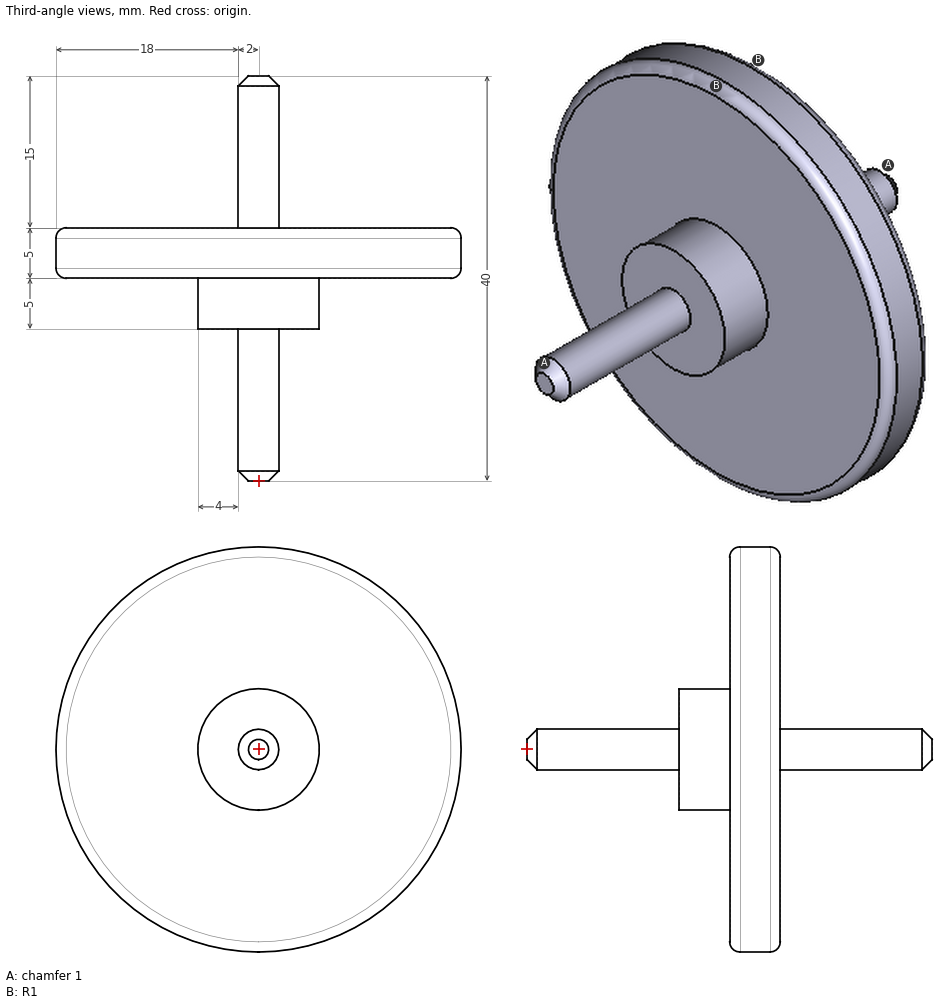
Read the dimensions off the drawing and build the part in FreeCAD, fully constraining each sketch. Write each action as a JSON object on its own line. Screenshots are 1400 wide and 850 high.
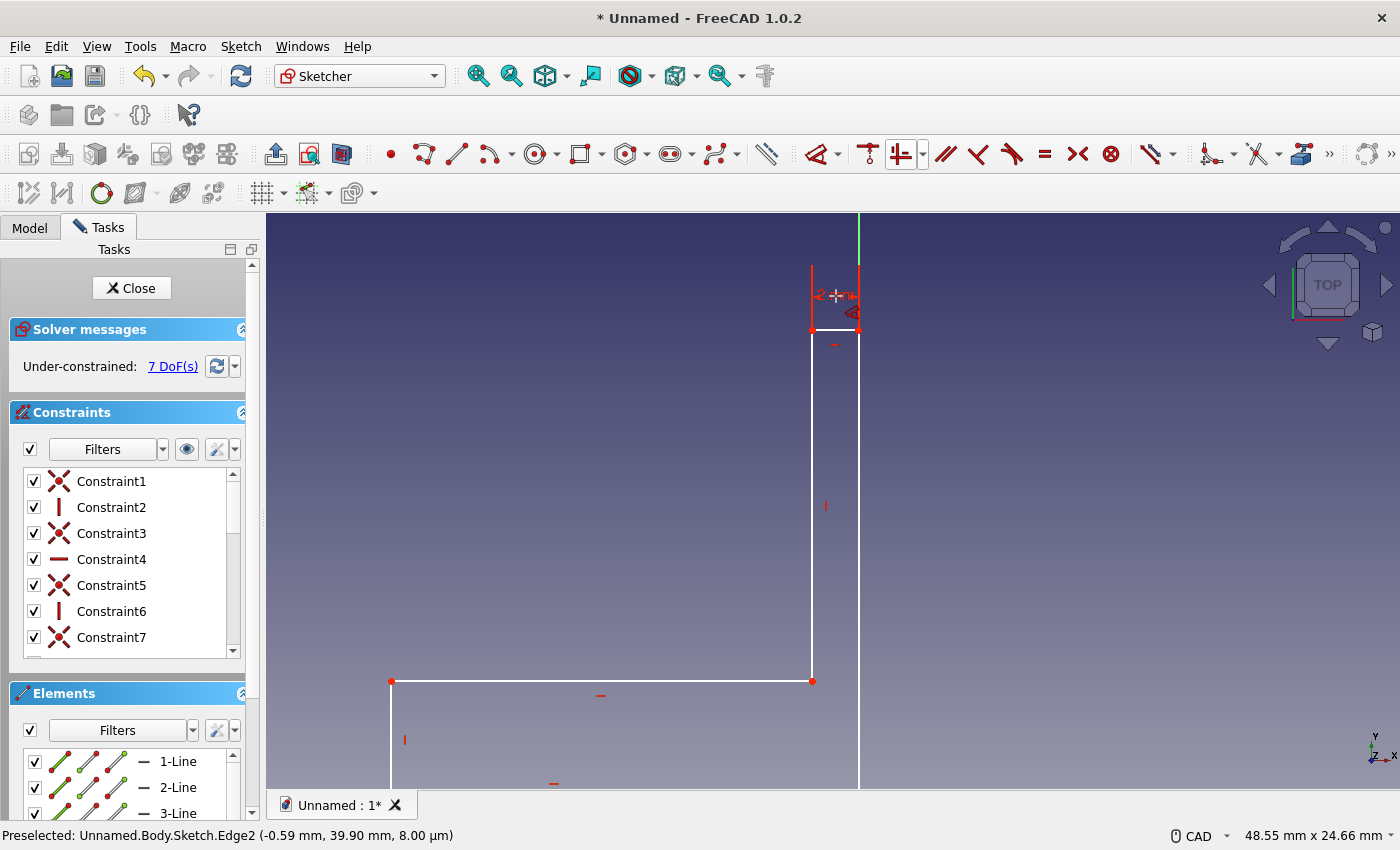
{"action": "left_click", "coordinate": [391, 716]}
{"action": "left_click", "coordinate": [357, 721]}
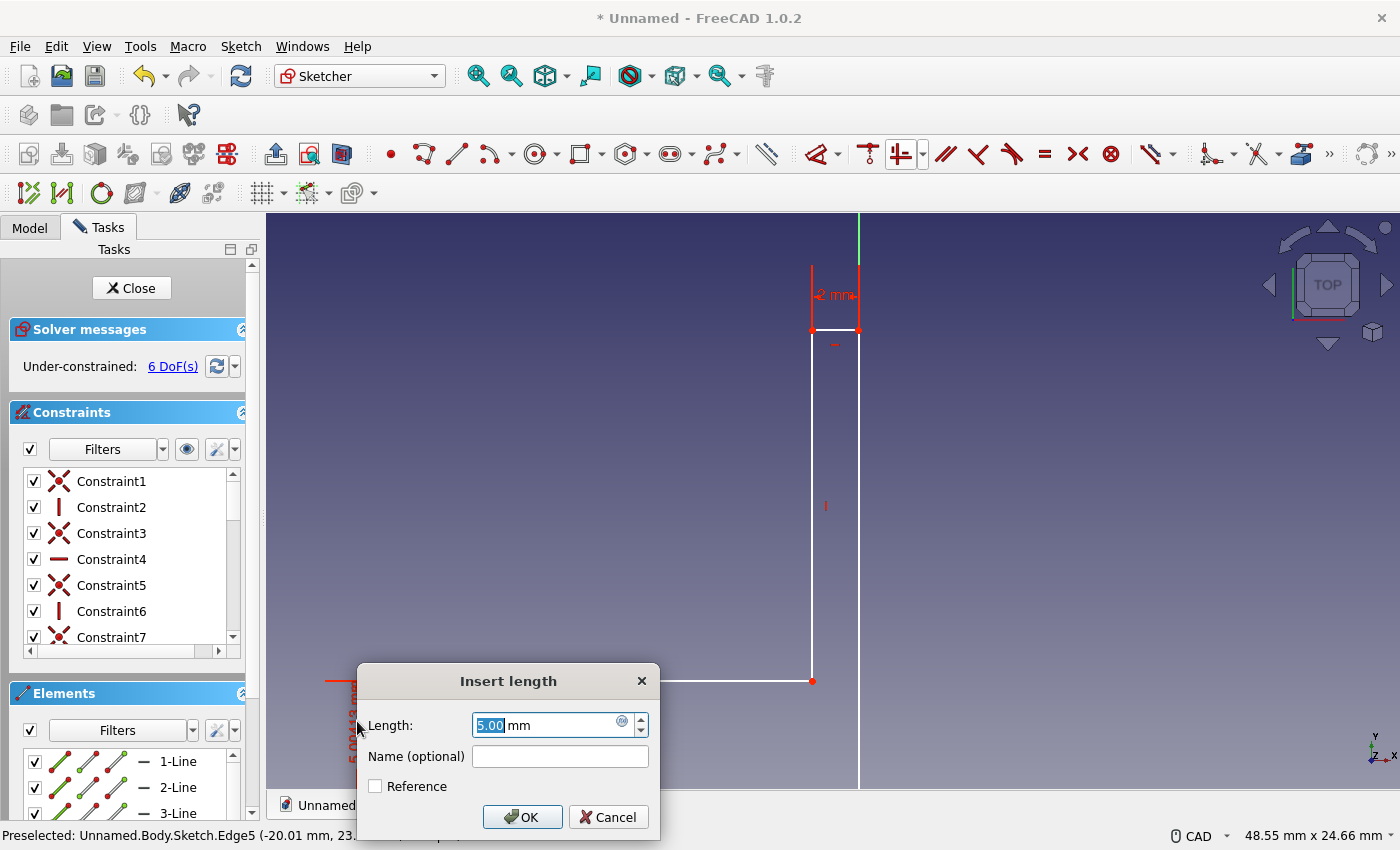
{"action": "type", "text": "5"}
{"action": "key", "text": "Return"}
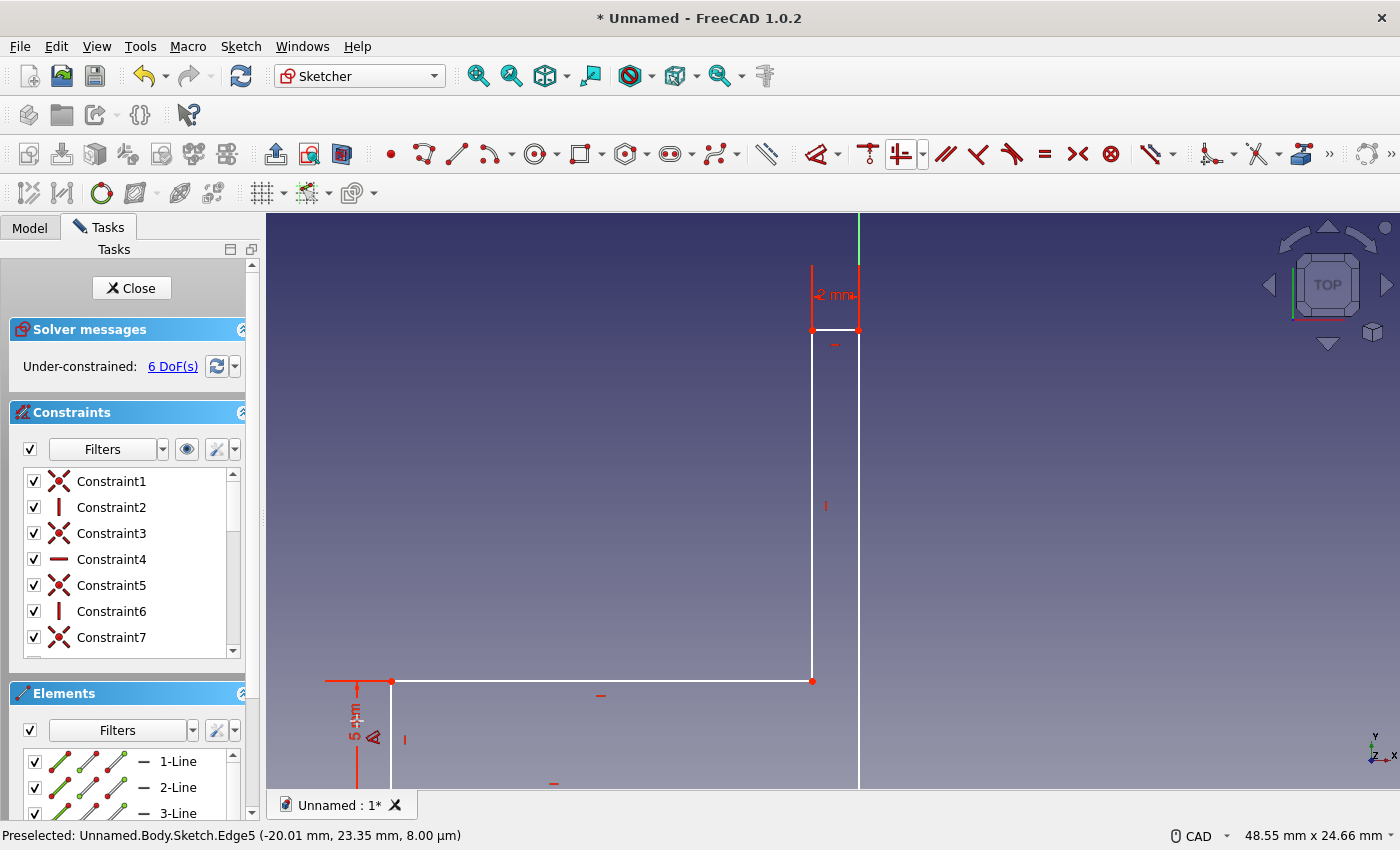
{"action": "scroll", "coordinate": [846, 330], "scroll_direction": "down", "scroll_amount": 5}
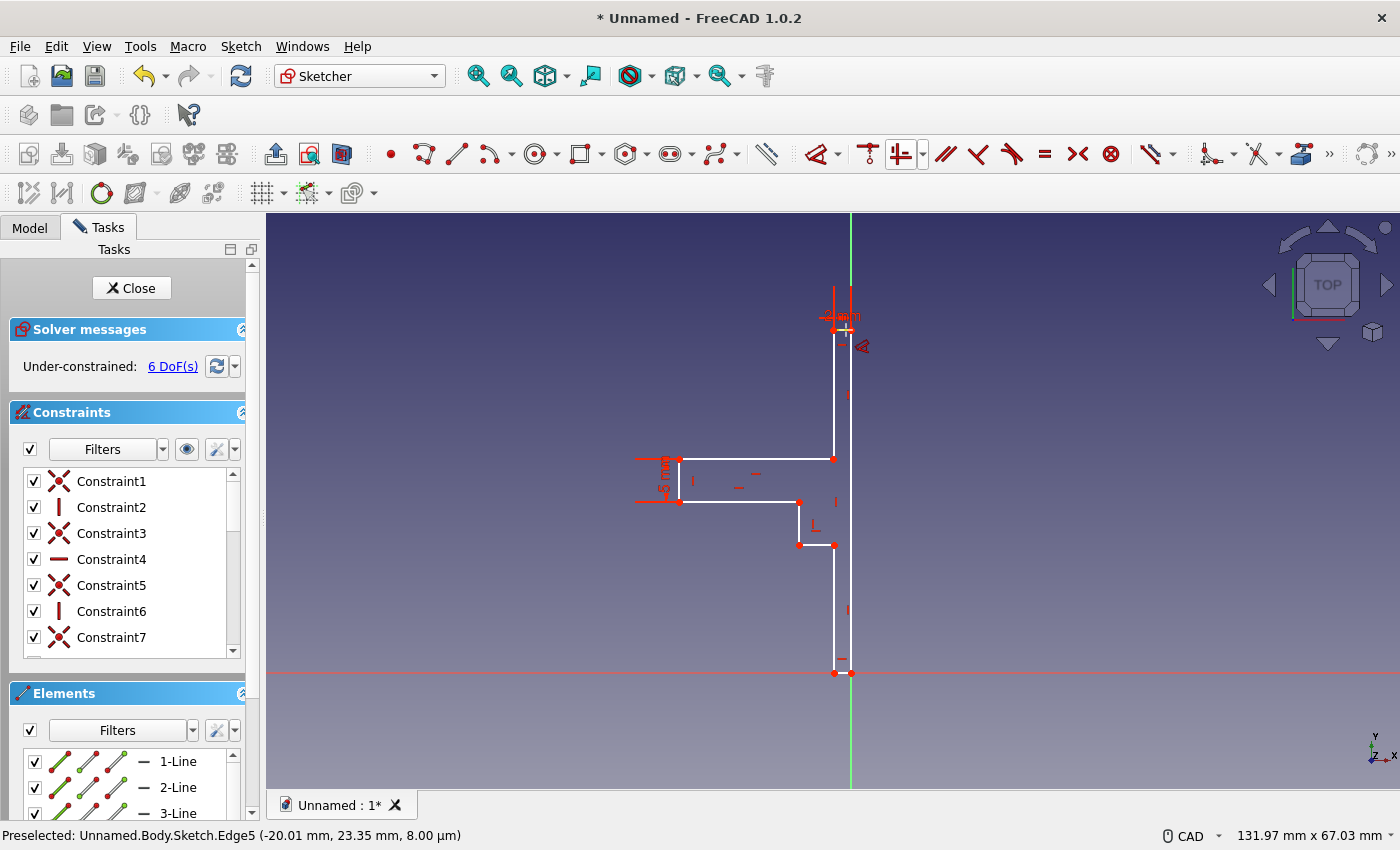
{"action": "left_click", "coordinate": [799, 515]}
{"action": "left_click", "coordinate": [833, 524]}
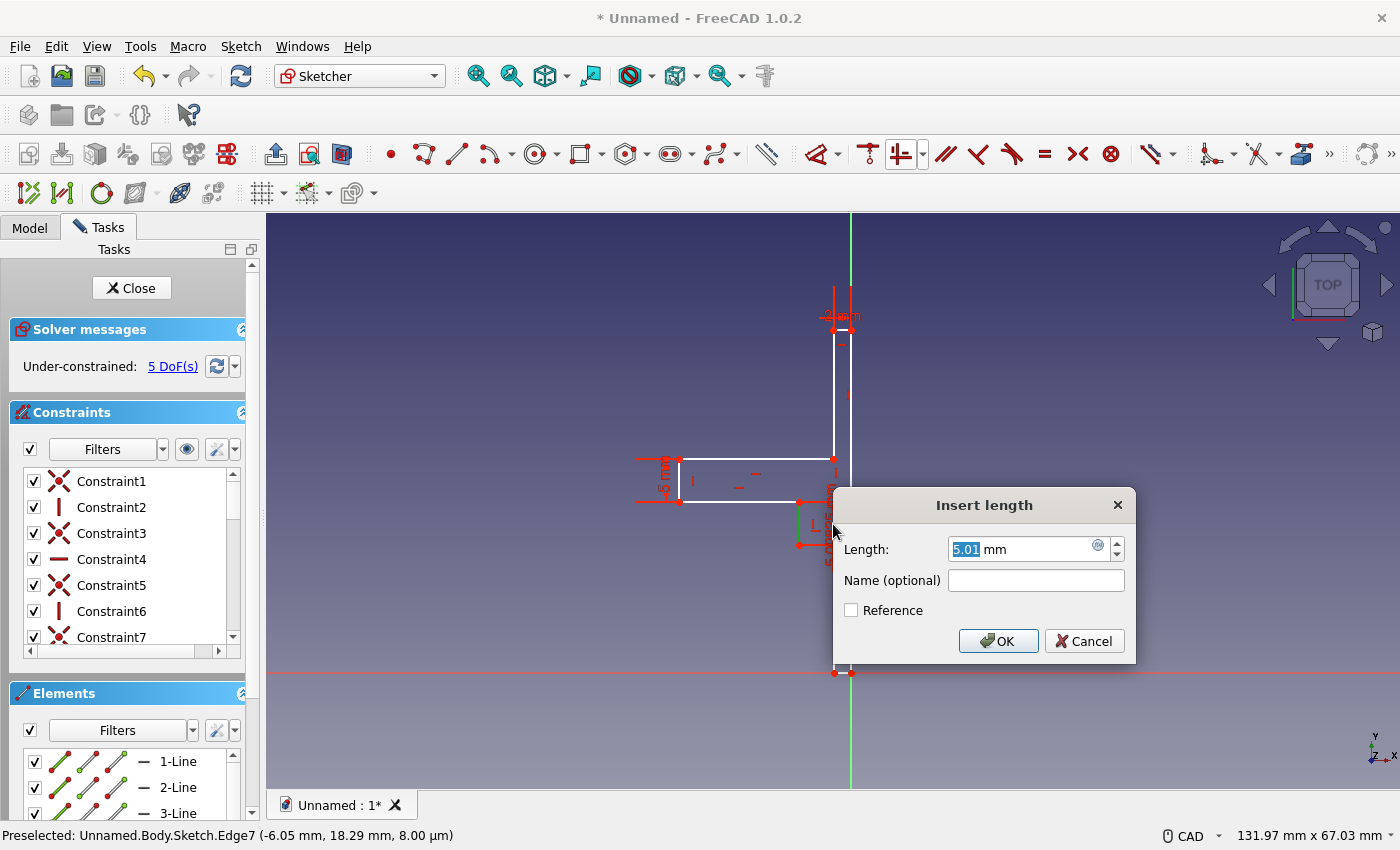
{"action": "type", "text": "5"}
{"action": "key", "text": "Return"}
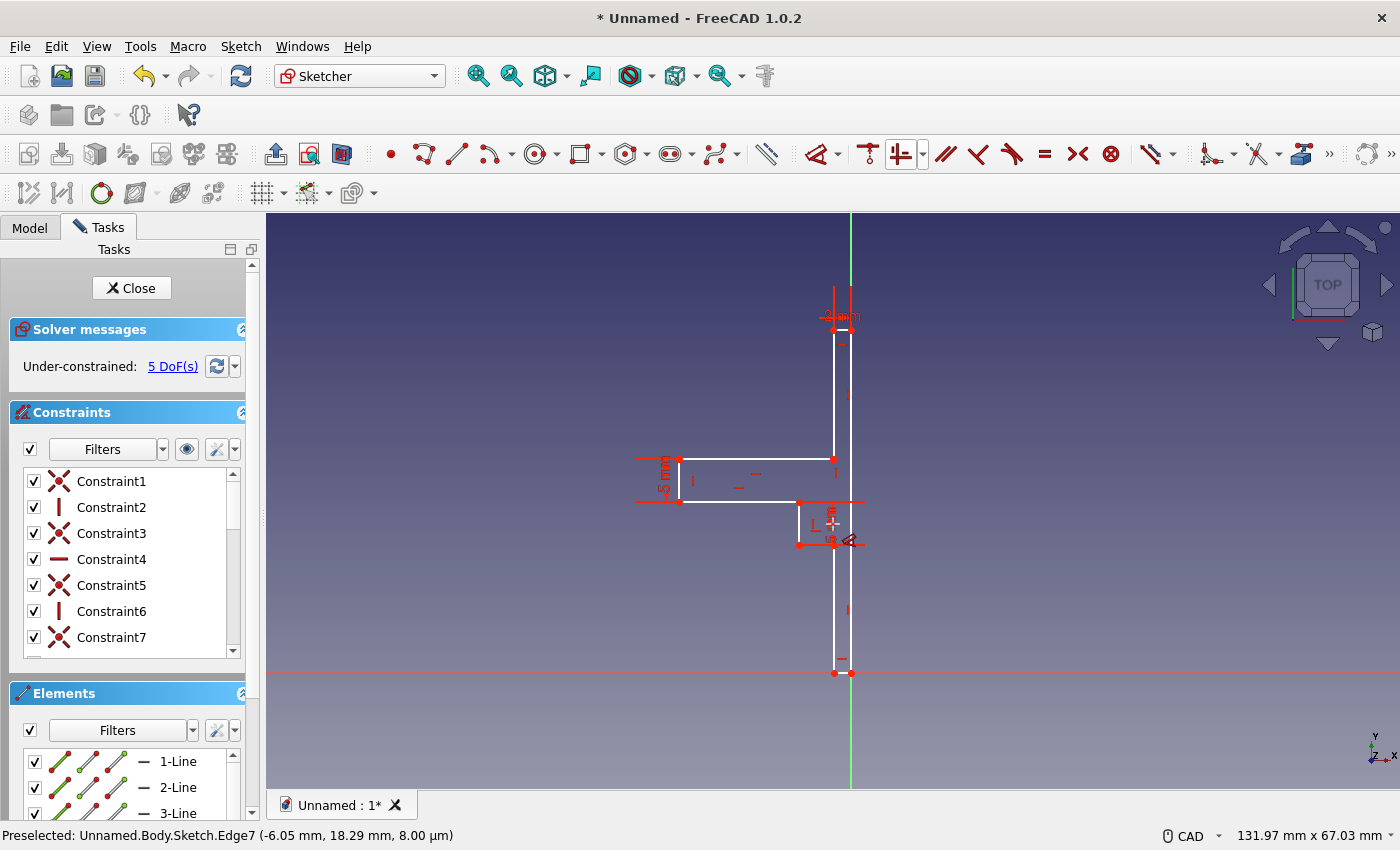
{"action": "scroll", "coordinate": [810, 545], "scroll_direction": "up", "scroll_amount": 2}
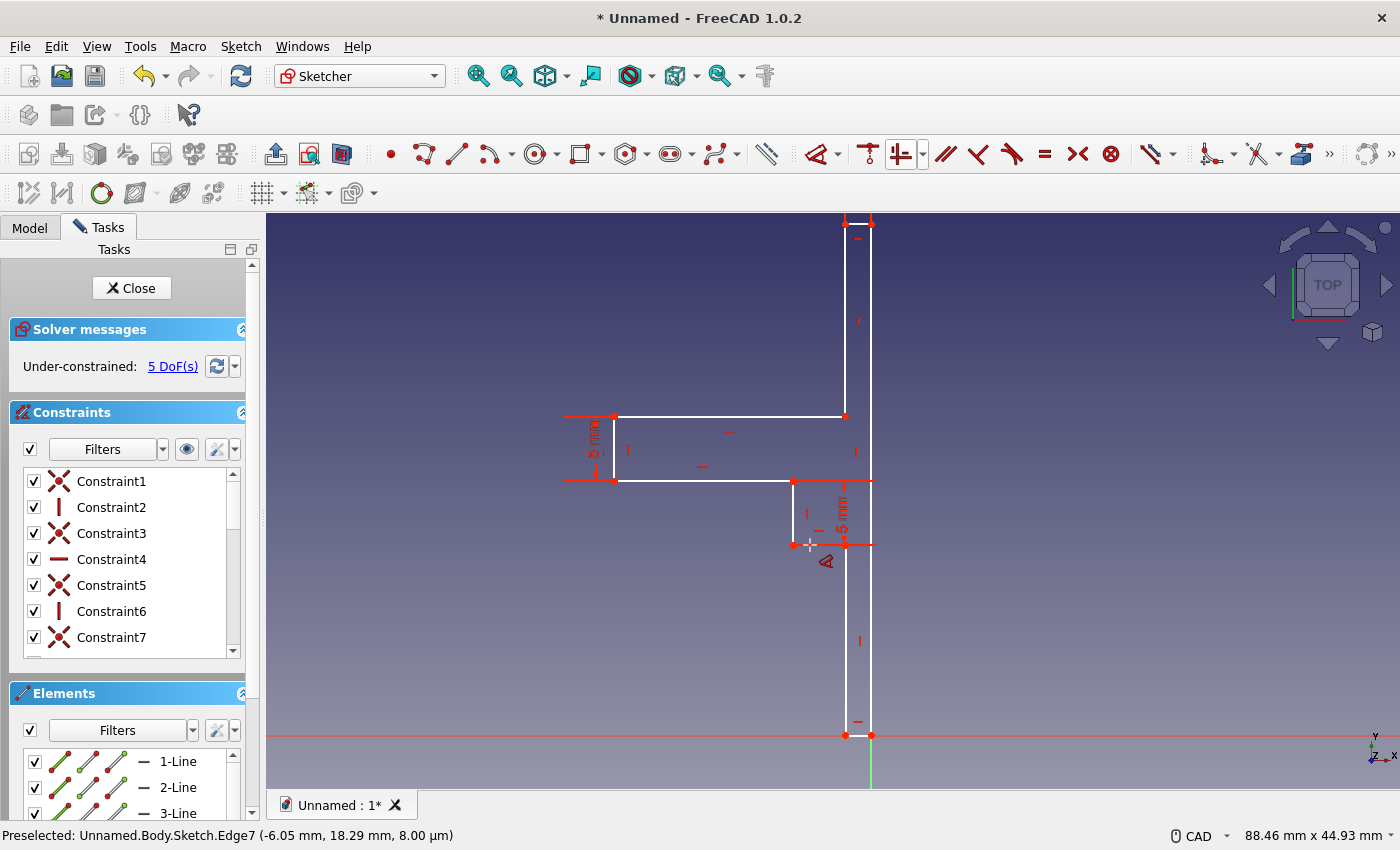
{"action": "left_click", "coordinate": [809, 545]}
{"action": "left_click", "coordinate": [820, 579]}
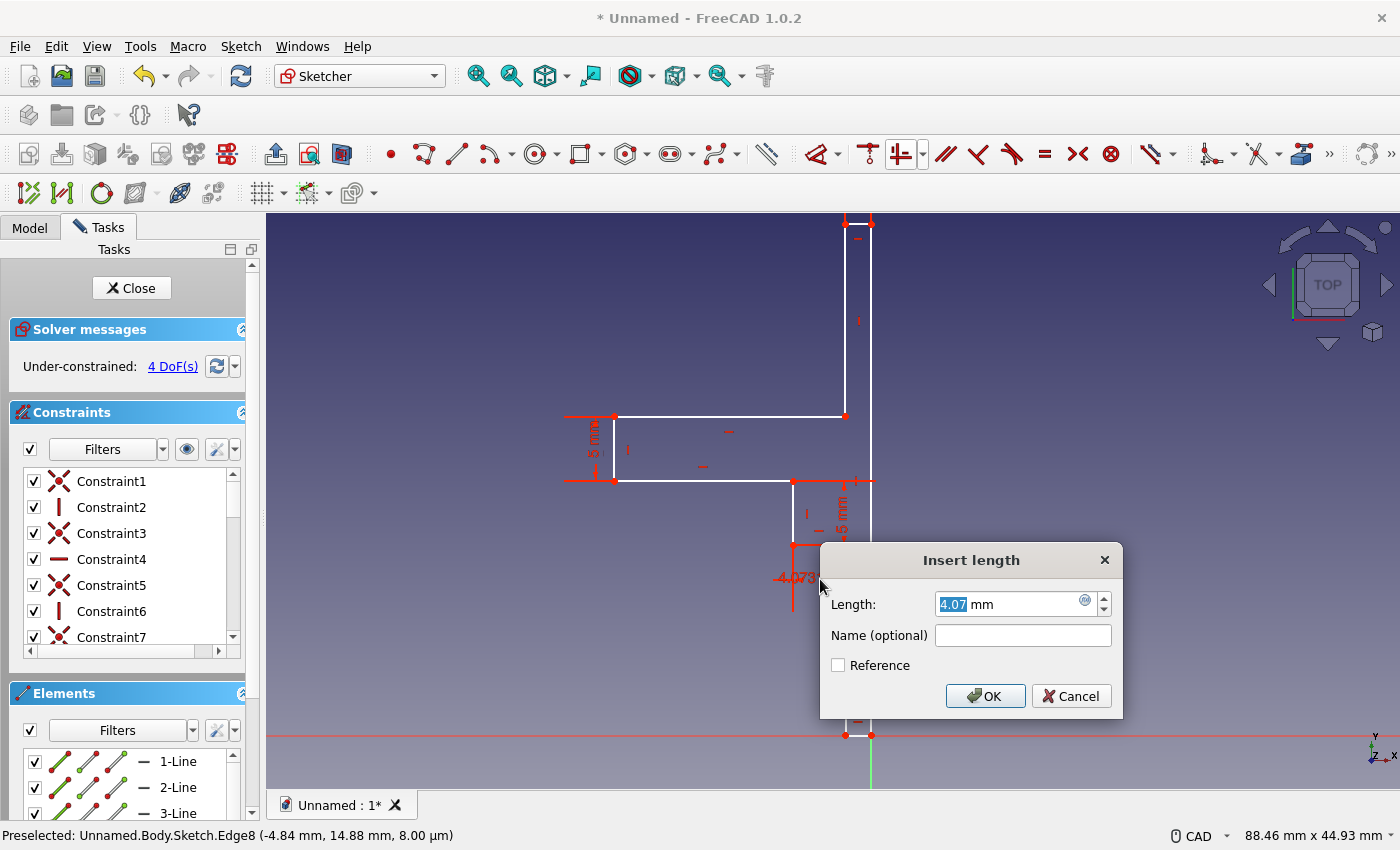
{"action": "type", "text": "4"}
{"action": "key", "text": "Return"}